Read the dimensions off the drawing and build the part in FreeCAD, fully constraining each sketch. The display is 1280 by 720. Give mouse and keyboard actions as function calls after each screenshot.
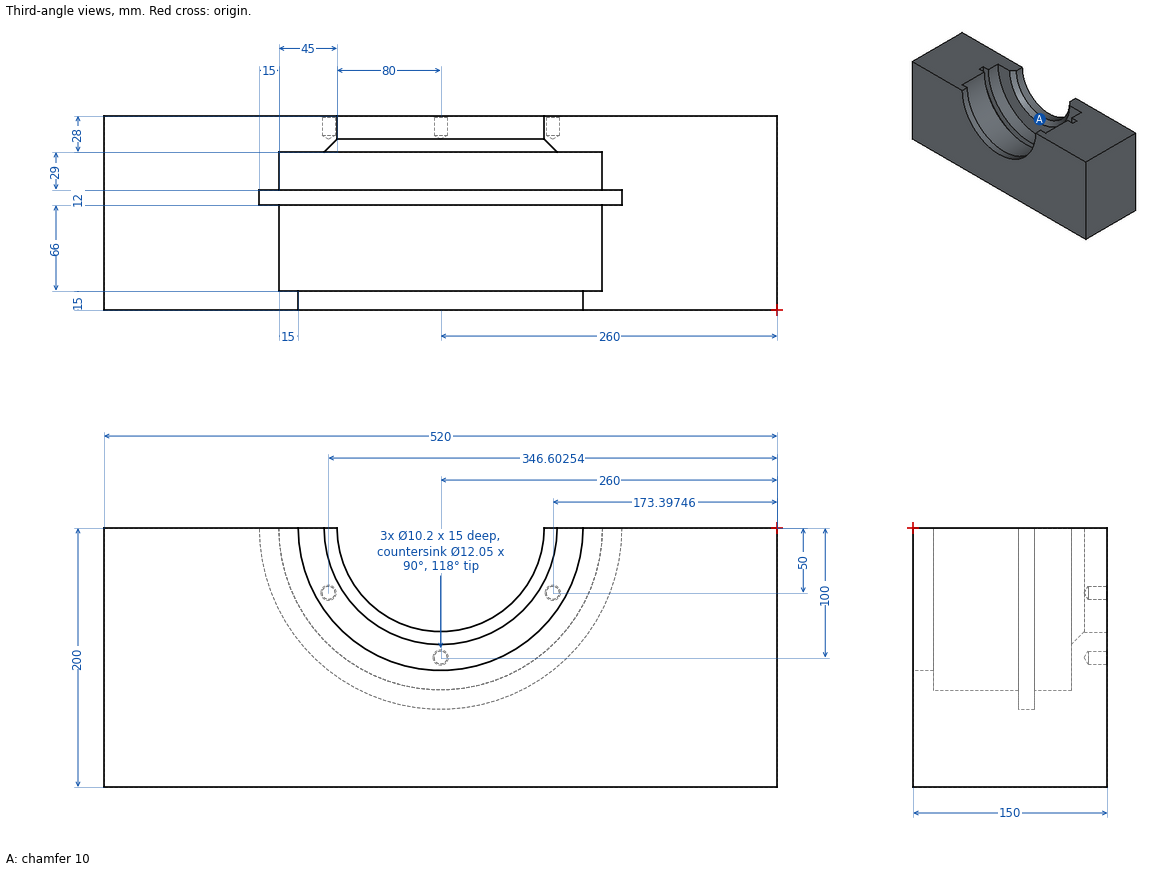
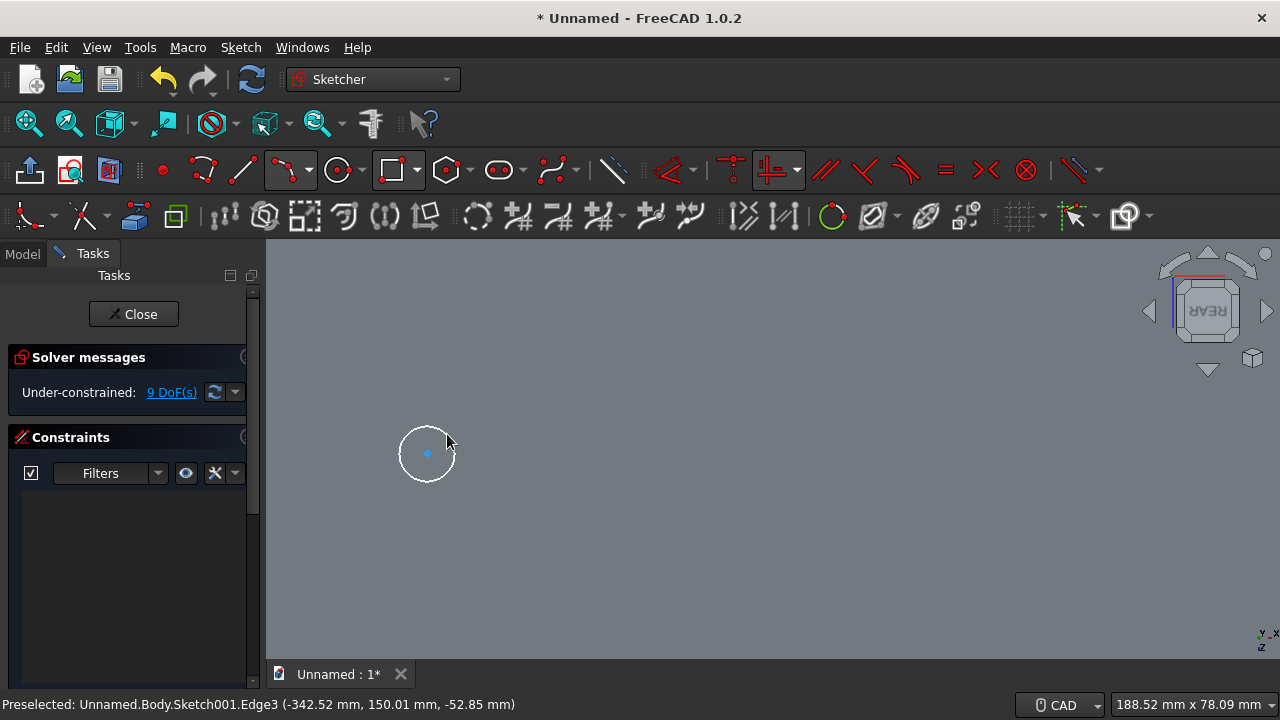
scroll(428, 453, down, 6)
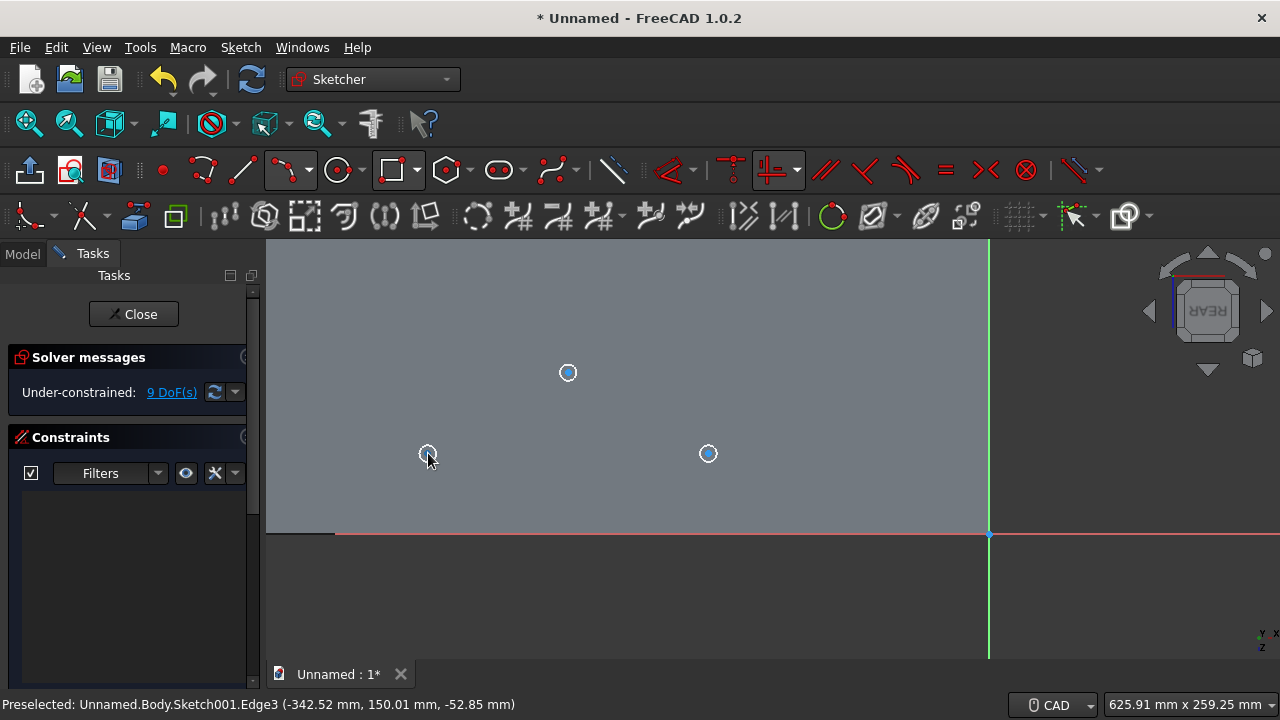
scroll(574, 367, up, 3)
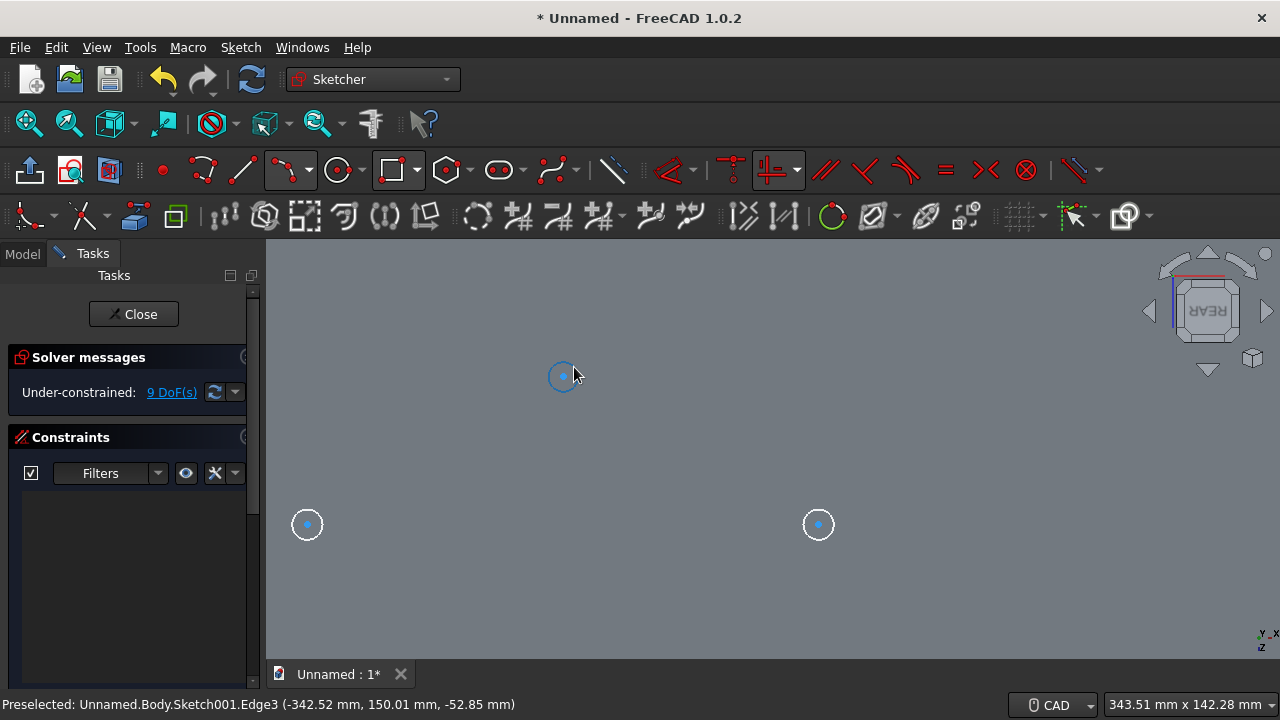
click(574, 367)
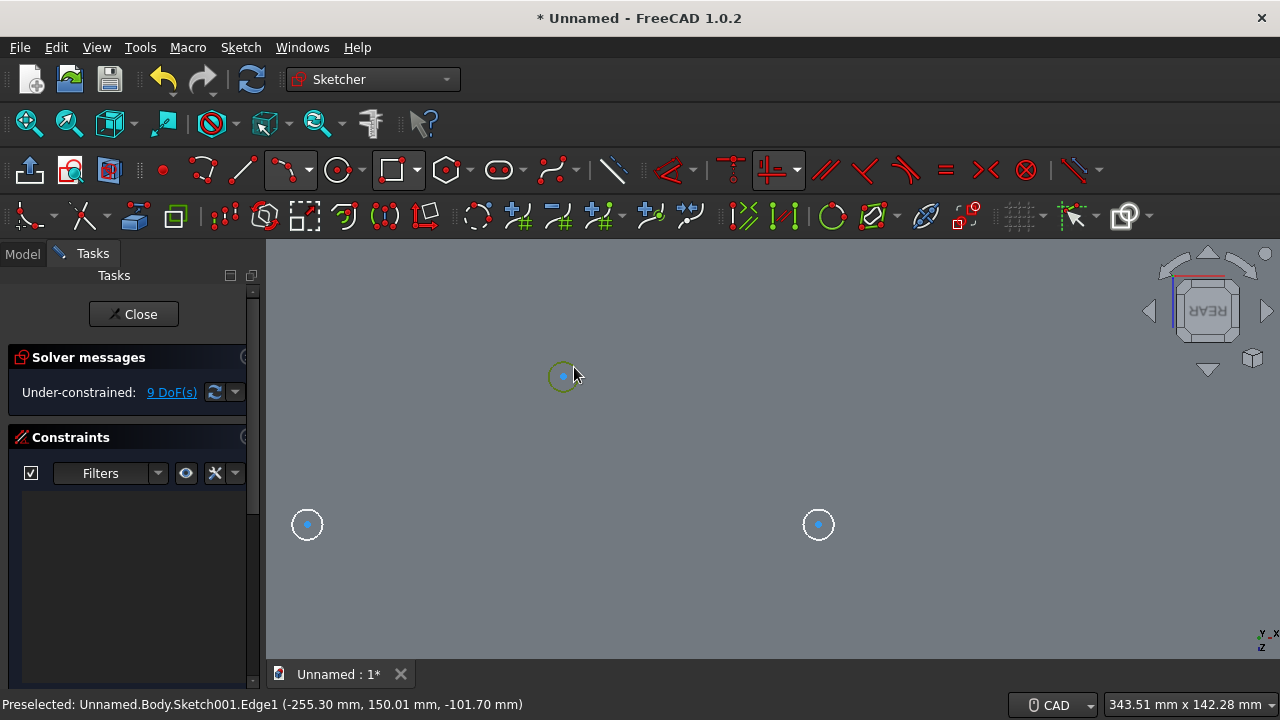
click(829, 514)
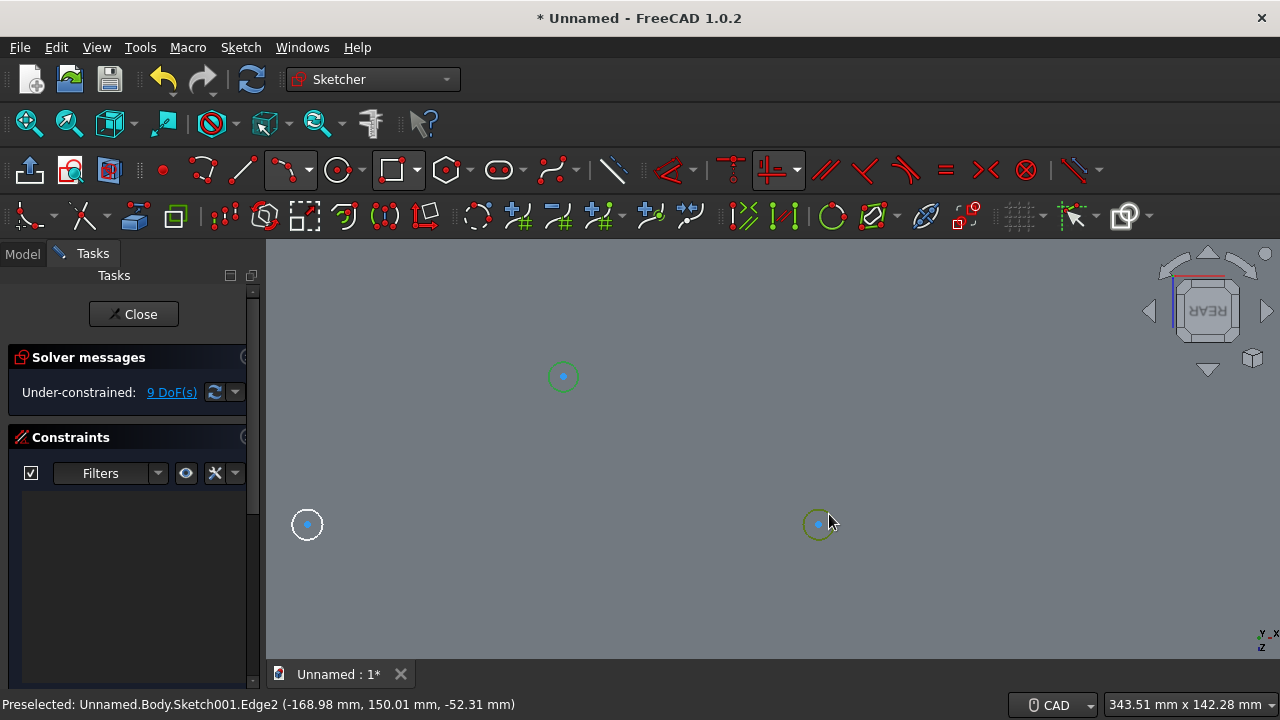
click(318, 514)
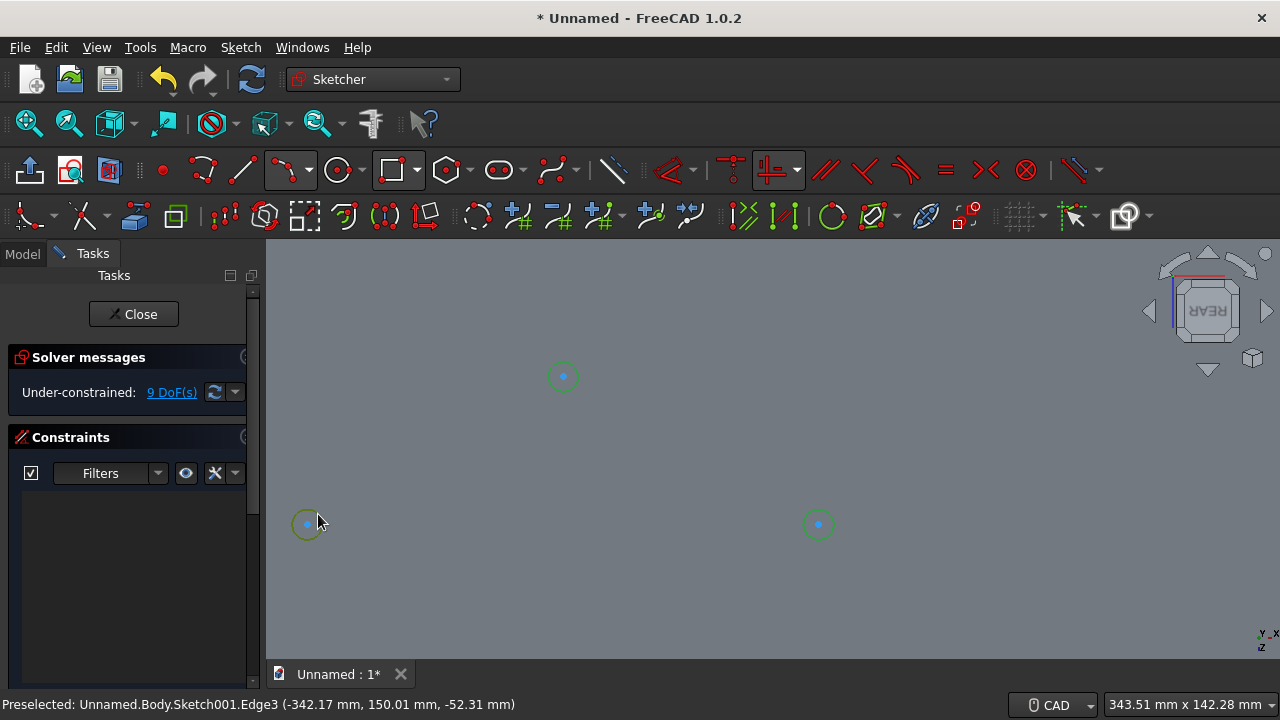
click(946, 170)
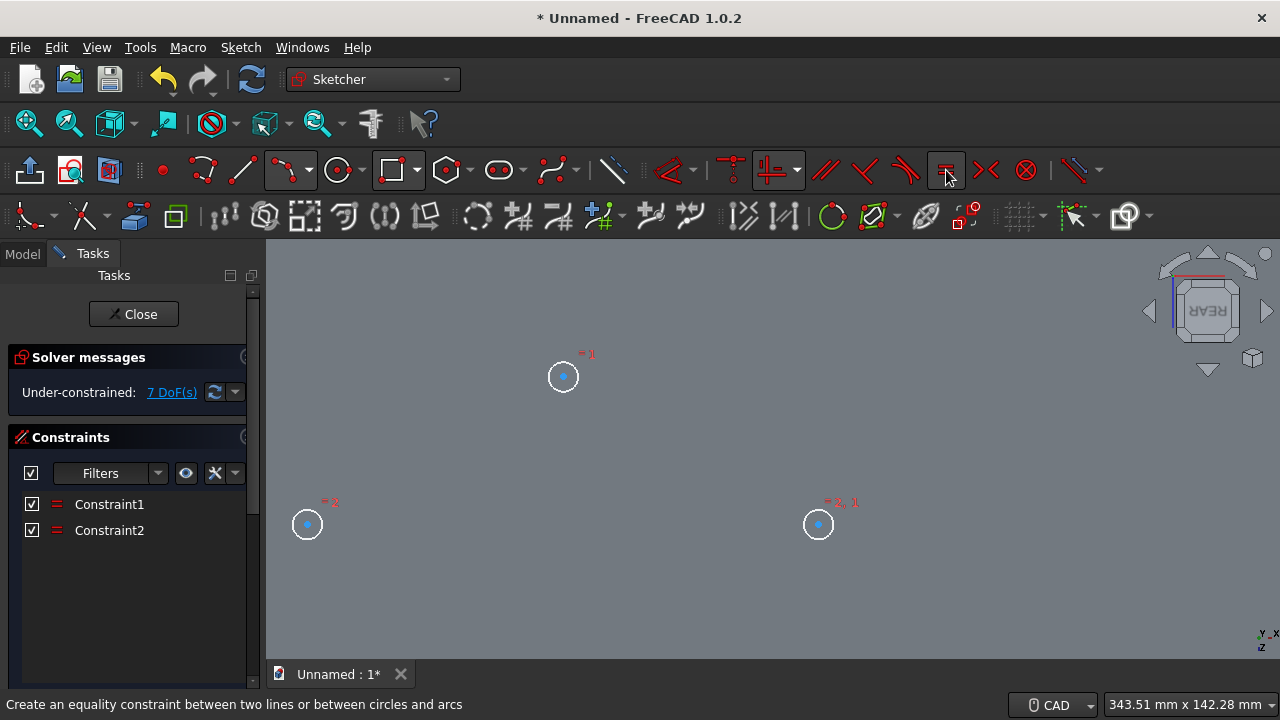
click(819, 525)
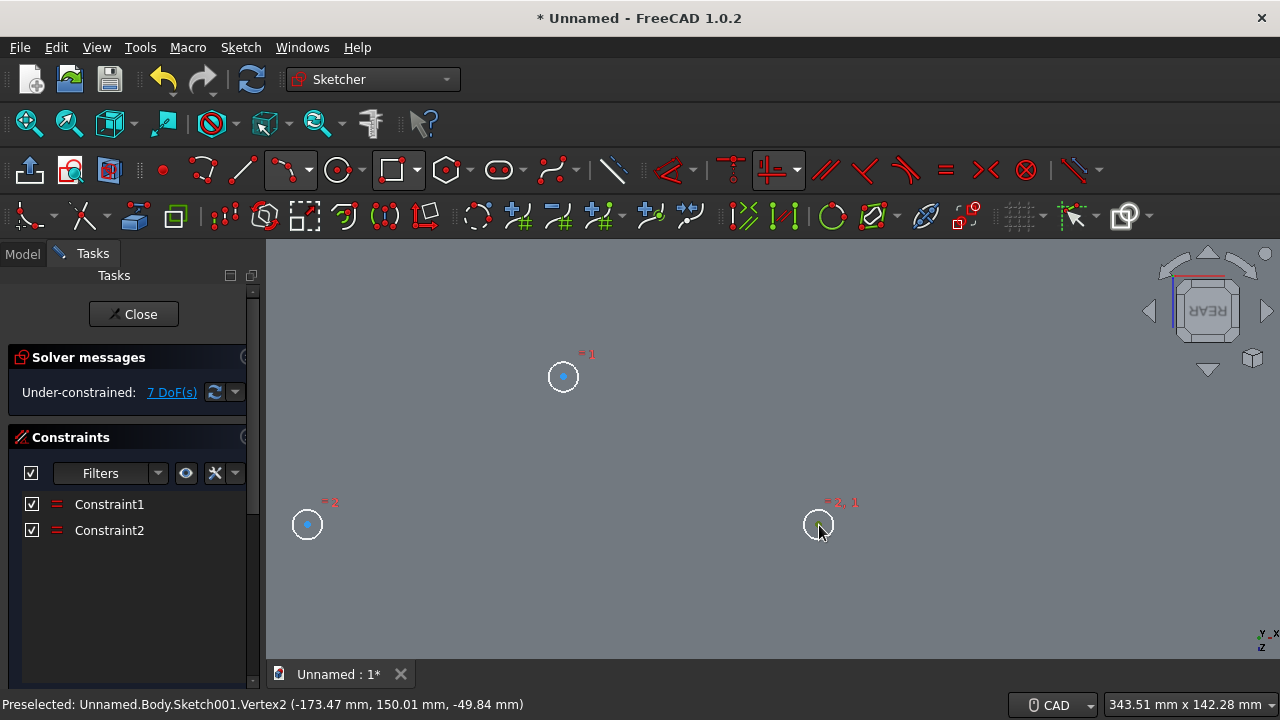
click(307, 525)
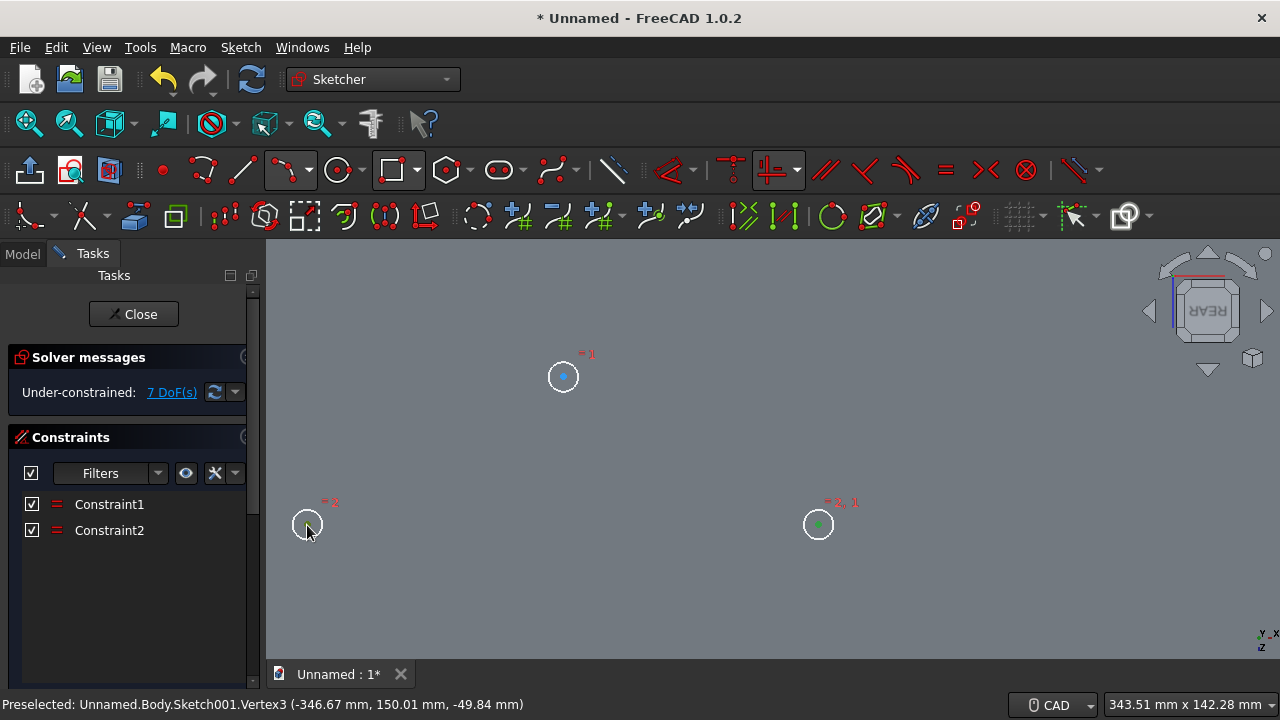
key(h)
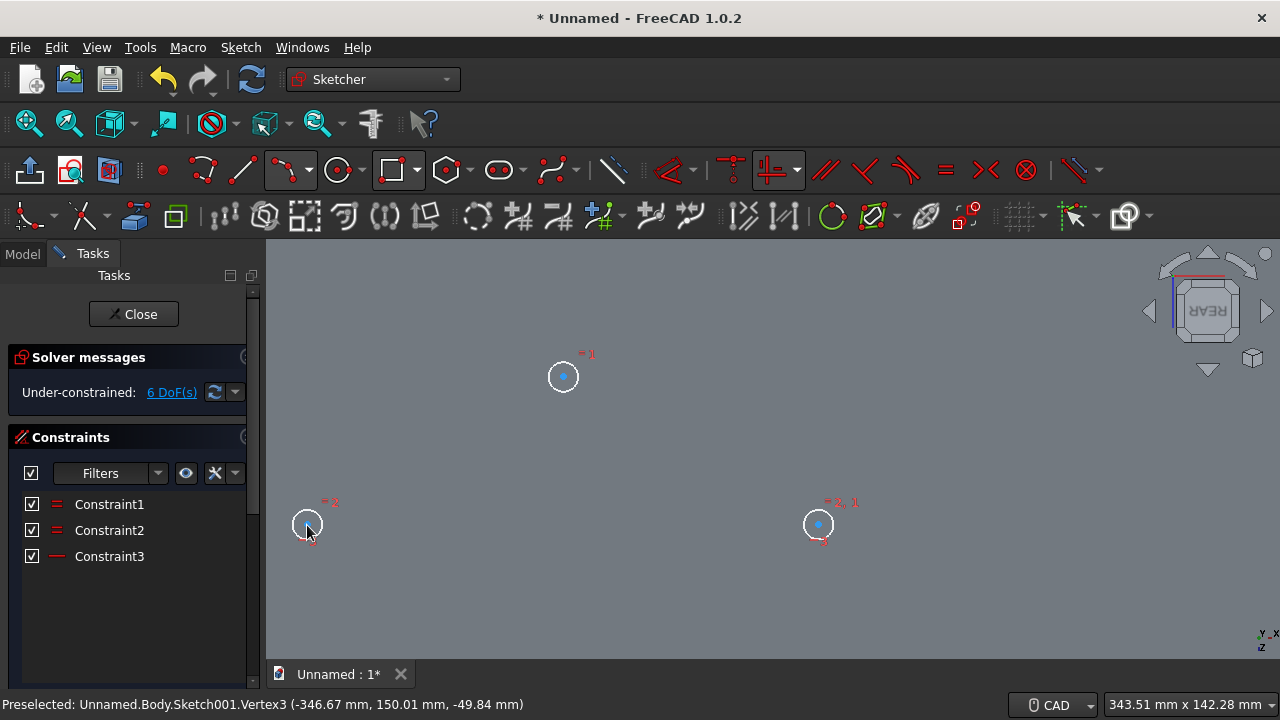
click(668, 170)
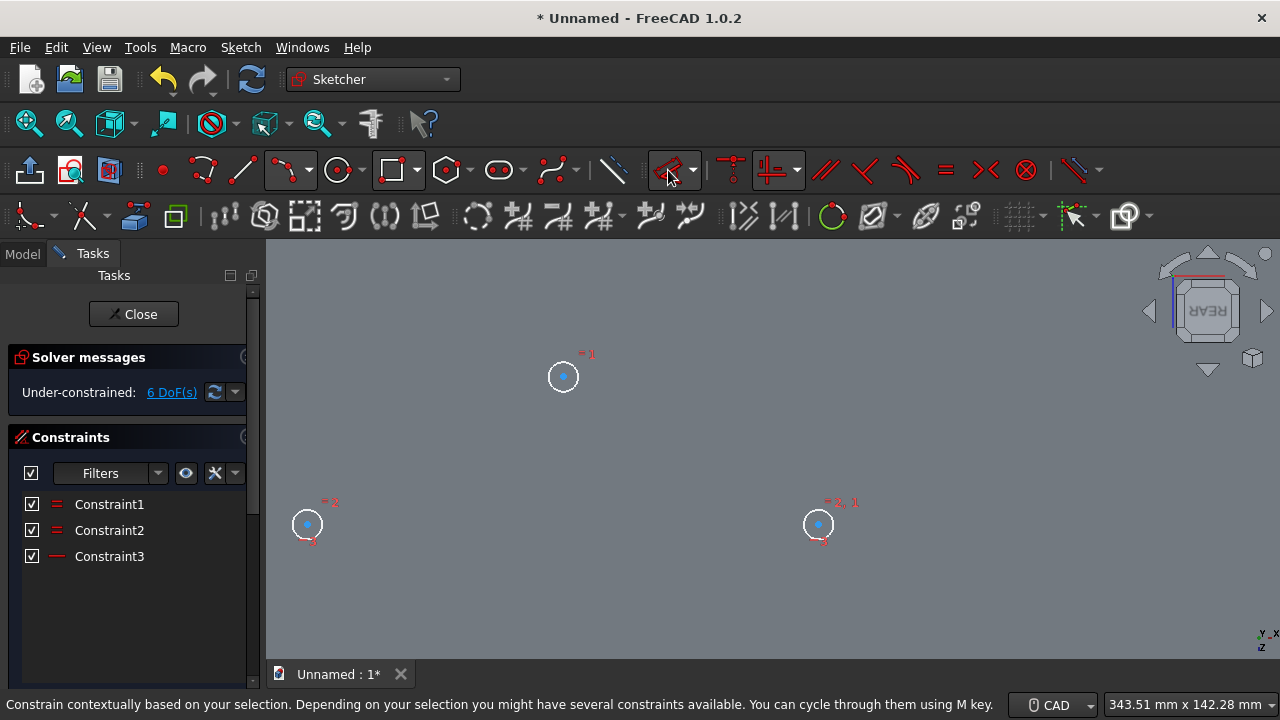
scroll(574, 367, up, 2)